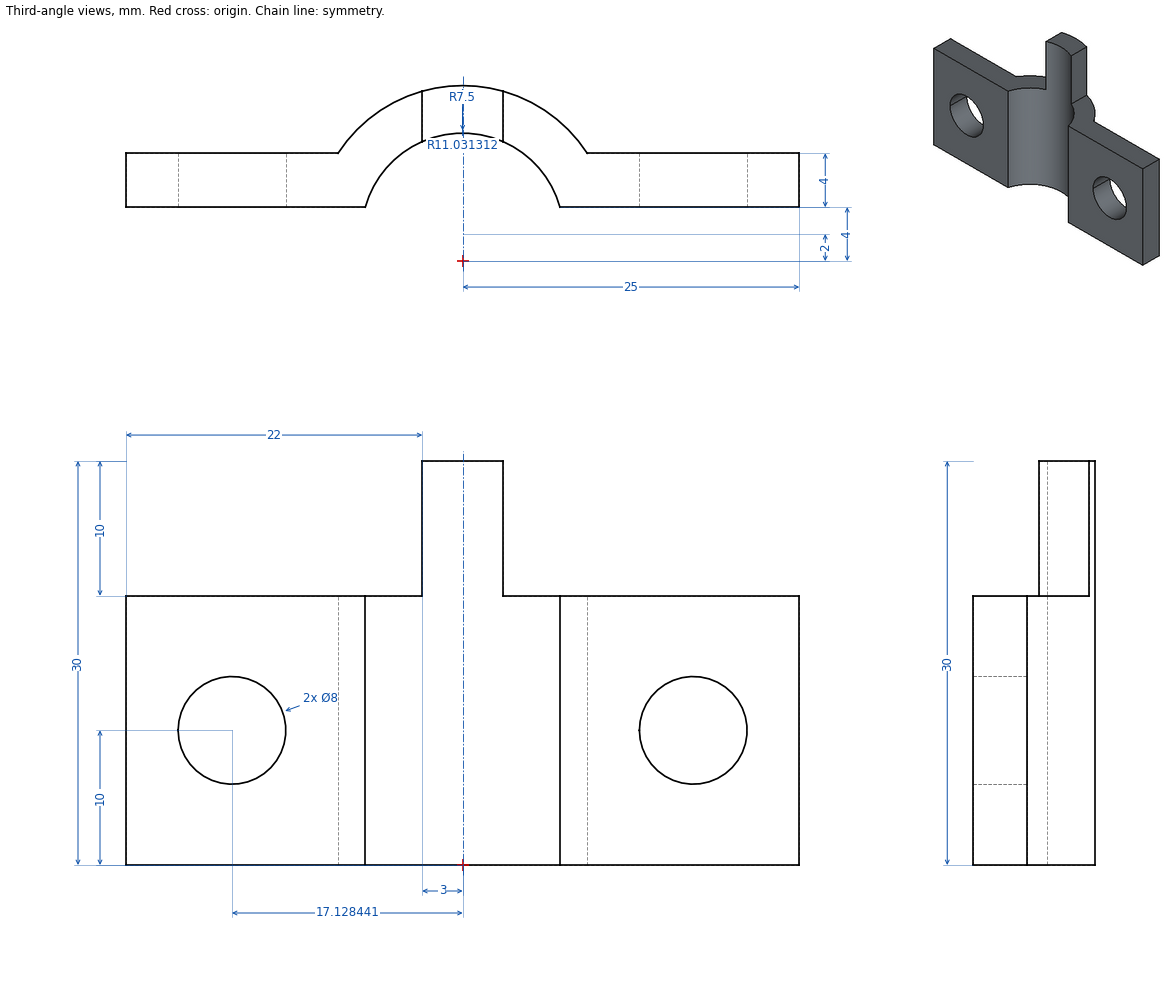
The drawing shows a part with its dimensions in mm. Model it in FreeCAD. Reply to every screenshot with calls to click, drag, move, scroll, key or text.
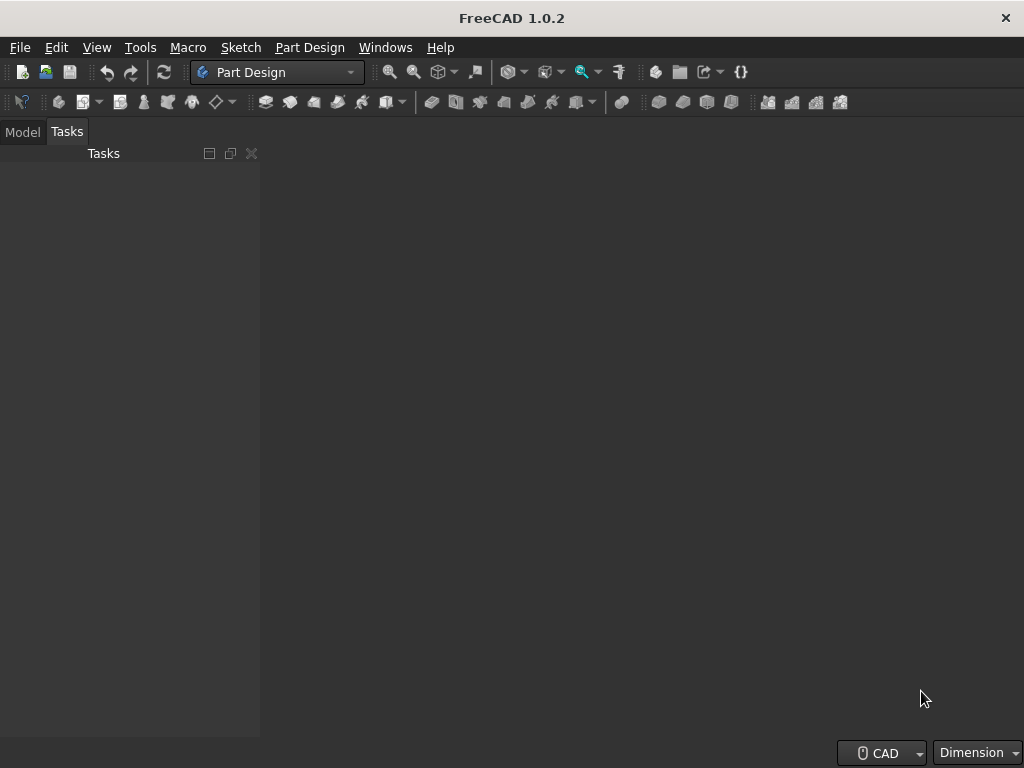
click(574, 102)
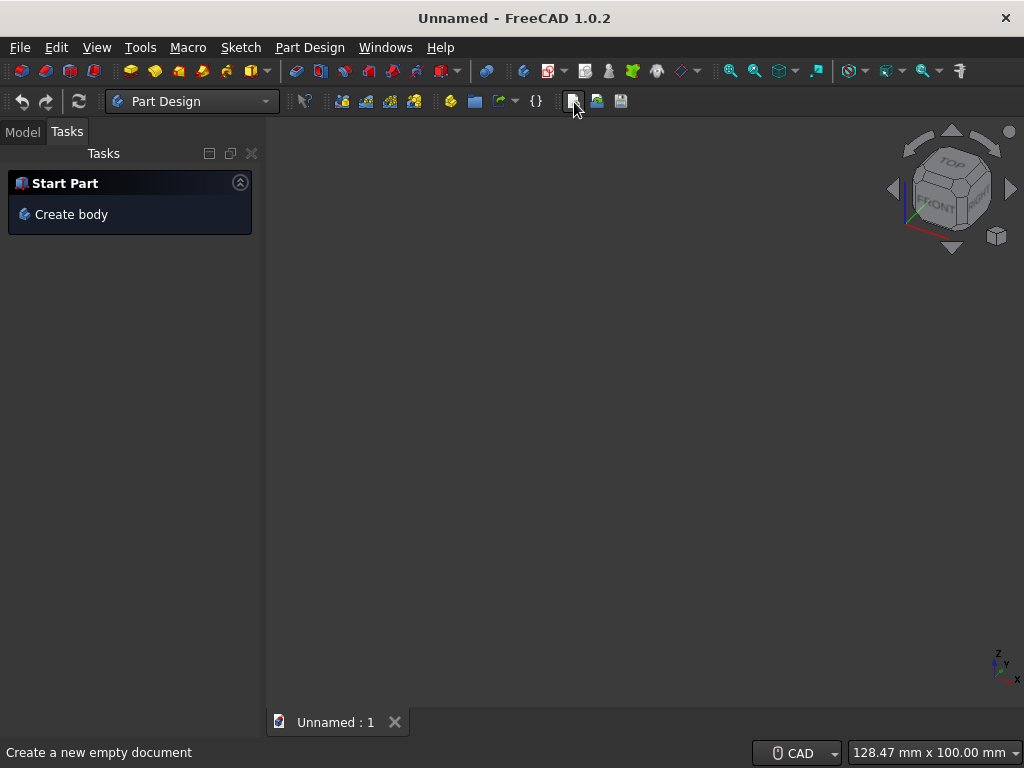
click(548, 72)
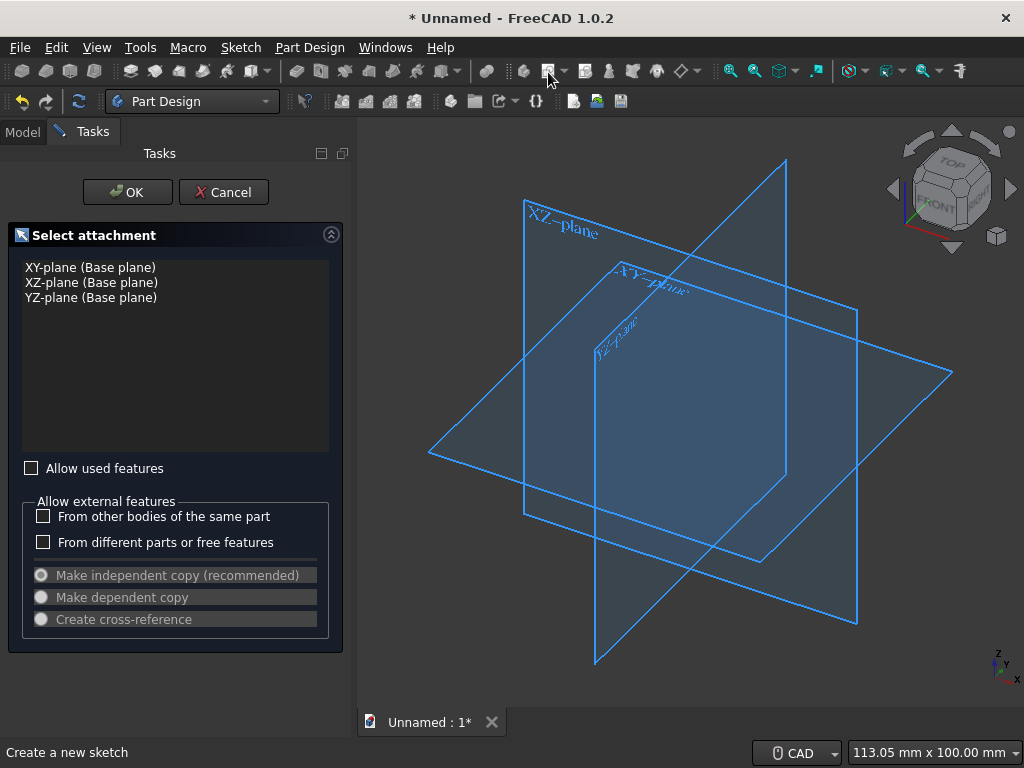
click(82, 268)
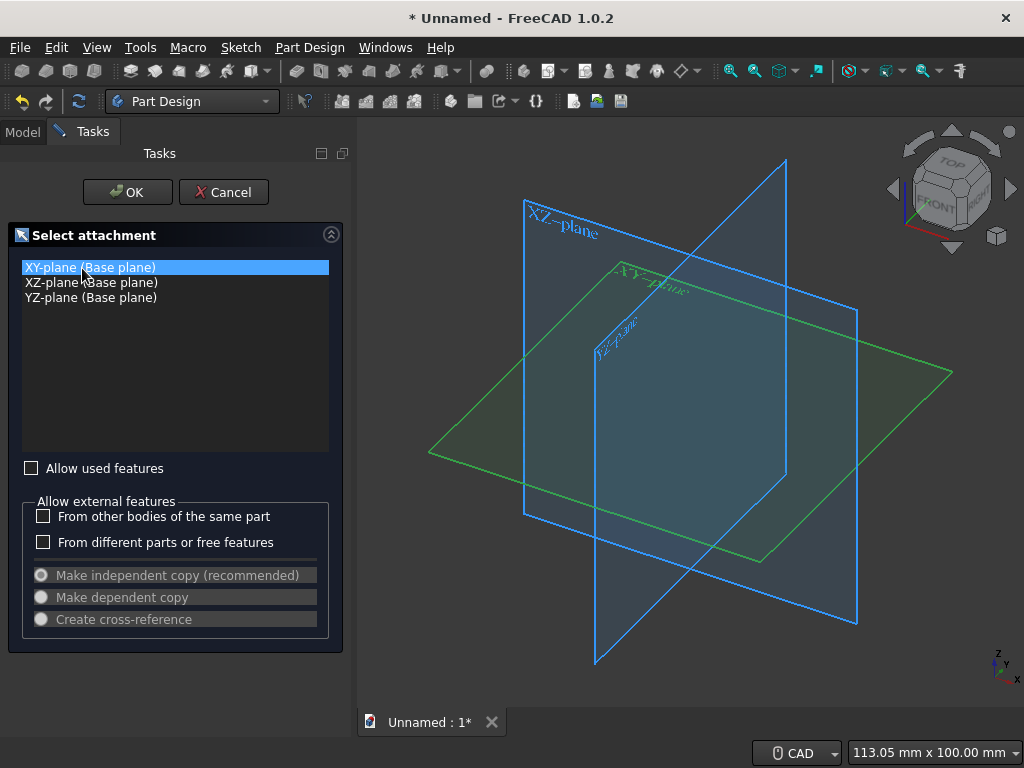
click(128, 192)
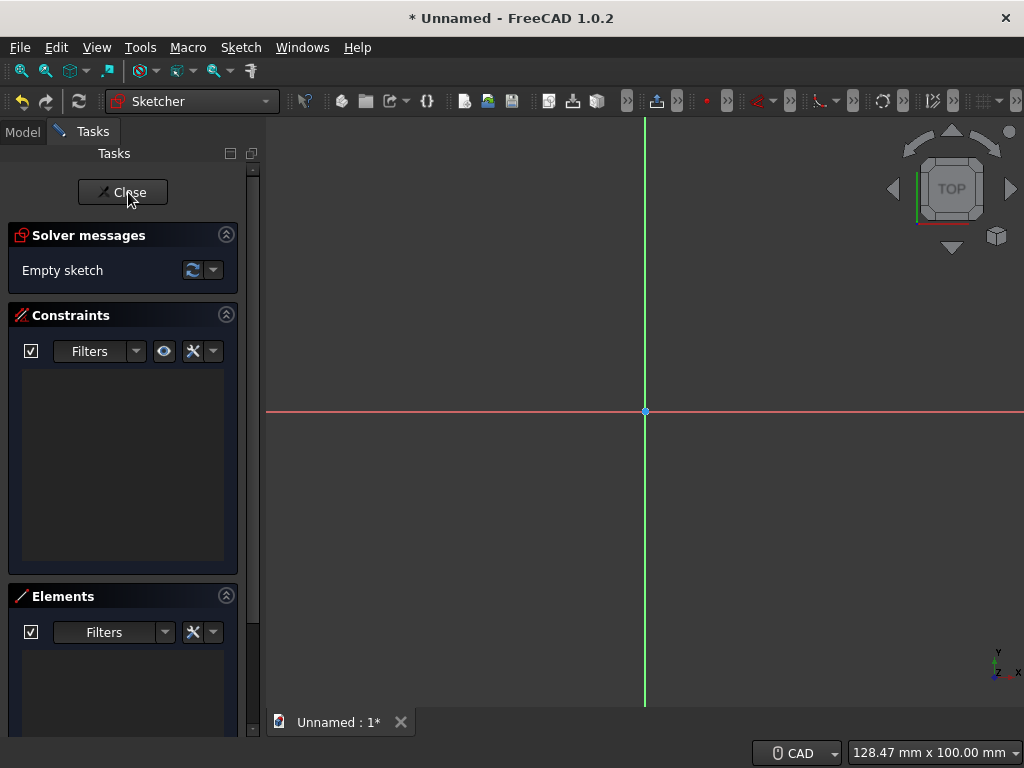
scroll(784, 295, up, 2)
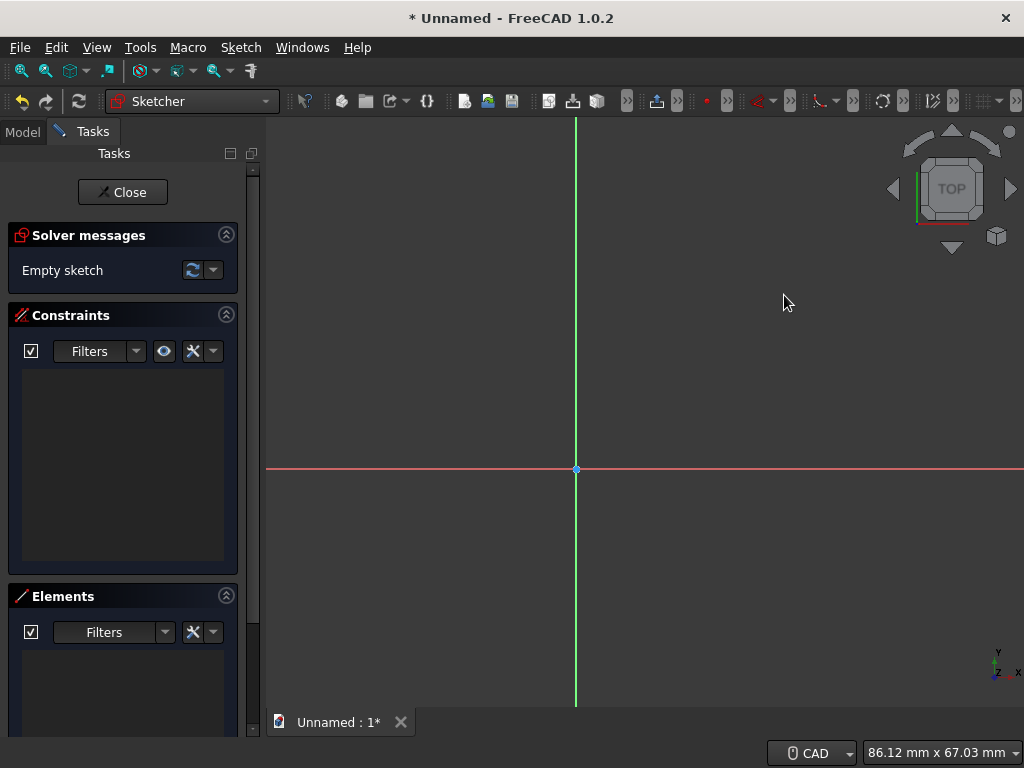
key(g)
key(m)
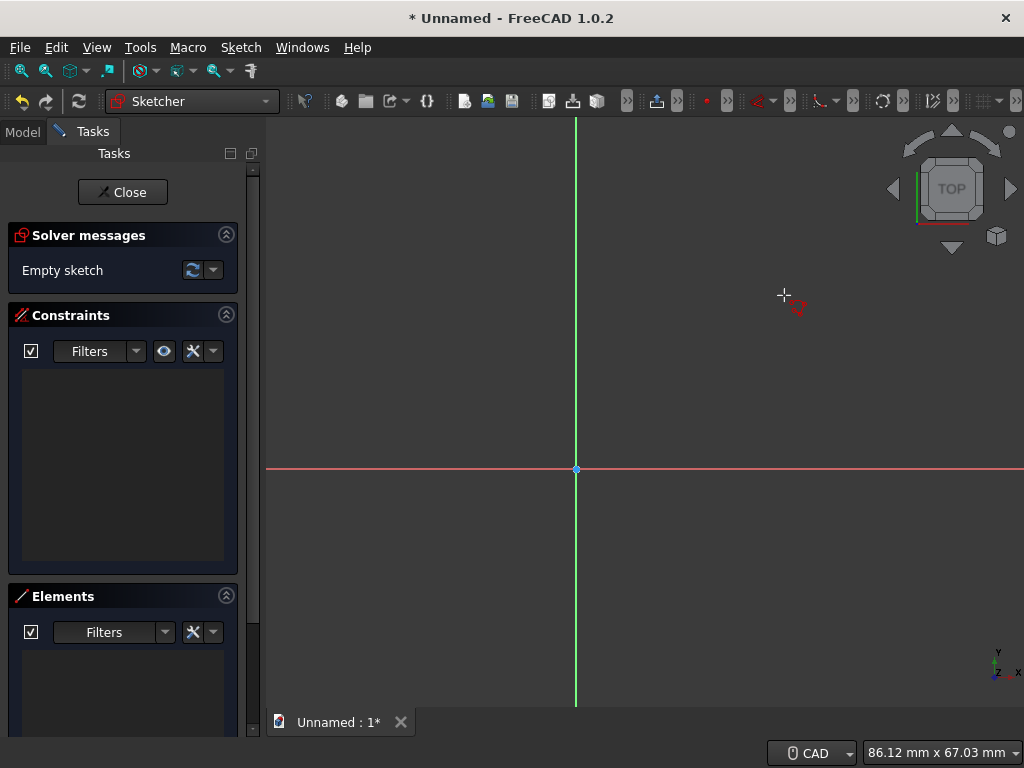
click(640, 434)
click(796, 434)
click(796, 399)
click(658, 399)
right_click(658, 399)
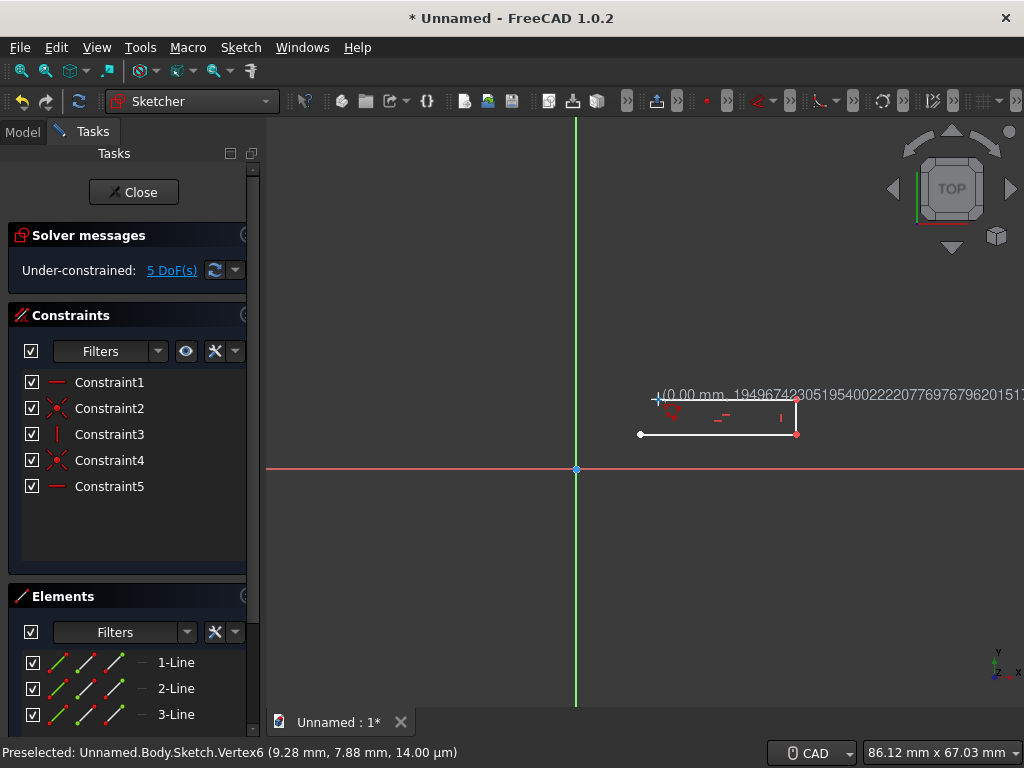
click(495, 399)
click(356, 399)
click(356, 434)
click(513, 434)
right_click(513, 434)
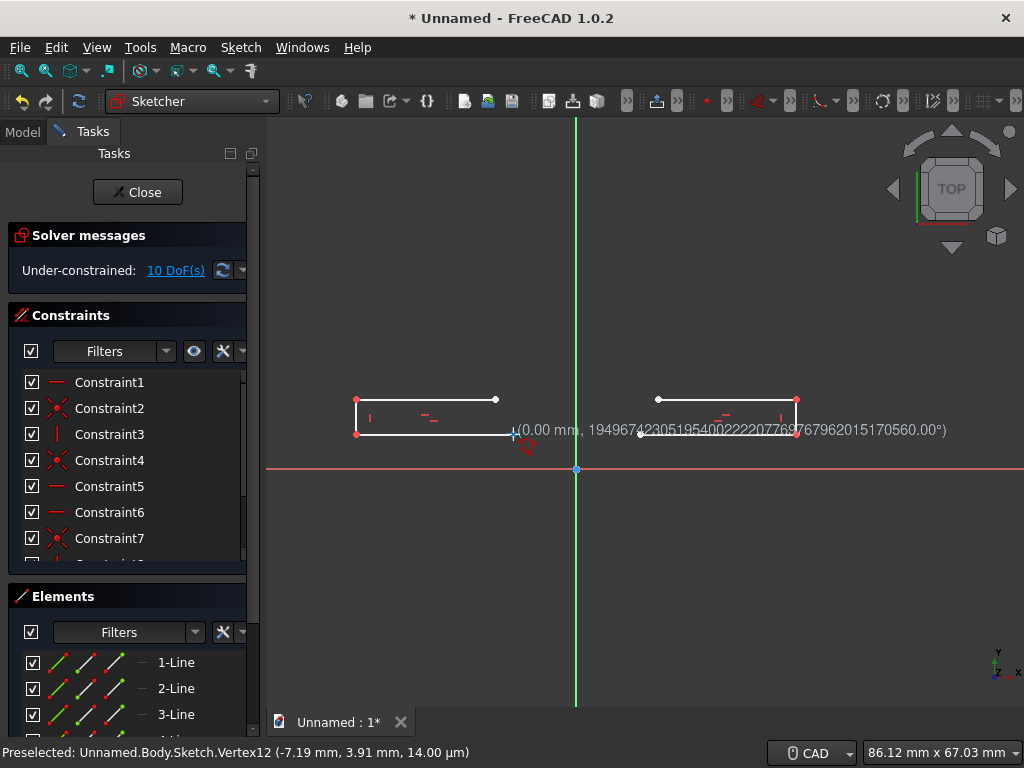
key(g)
key(3)
key(a)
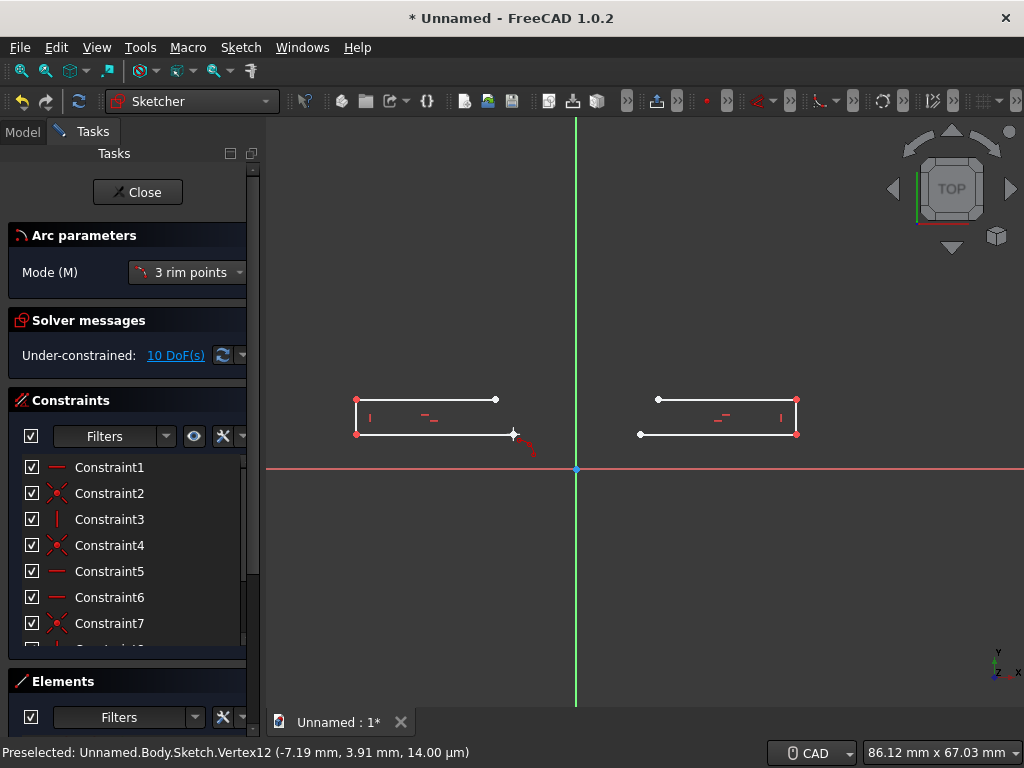
click(658, 400)
click(495, 400)
click(596, 357)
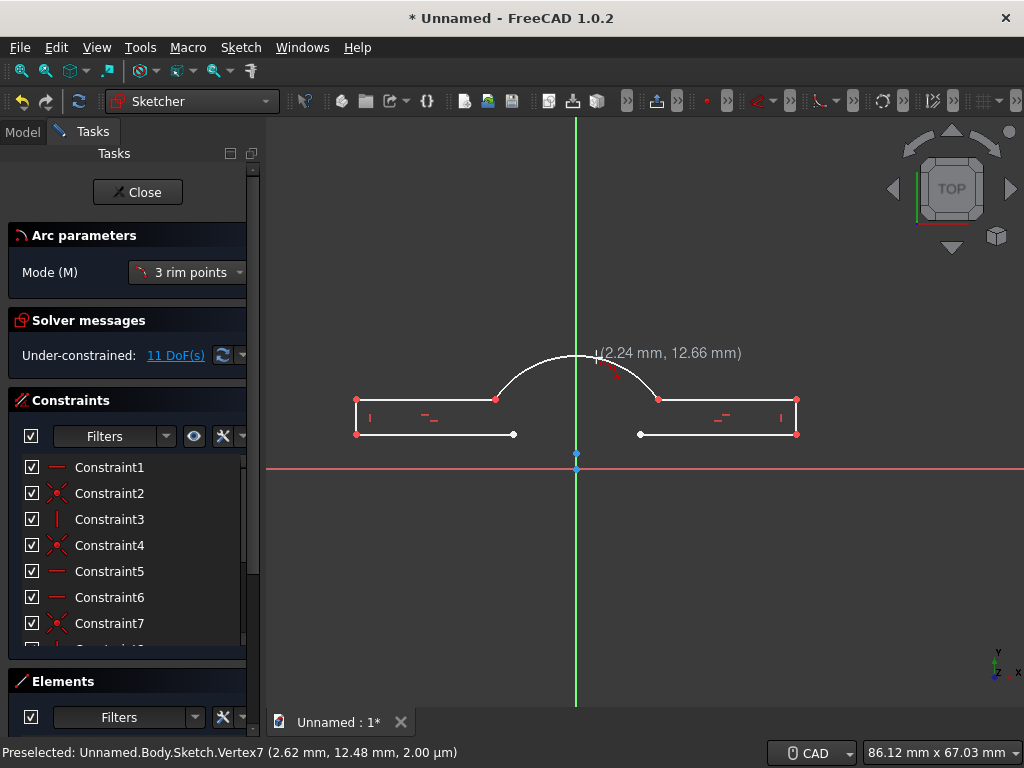
click(513, 435)
click(640, 435)
click(593, 388)
key(Escape)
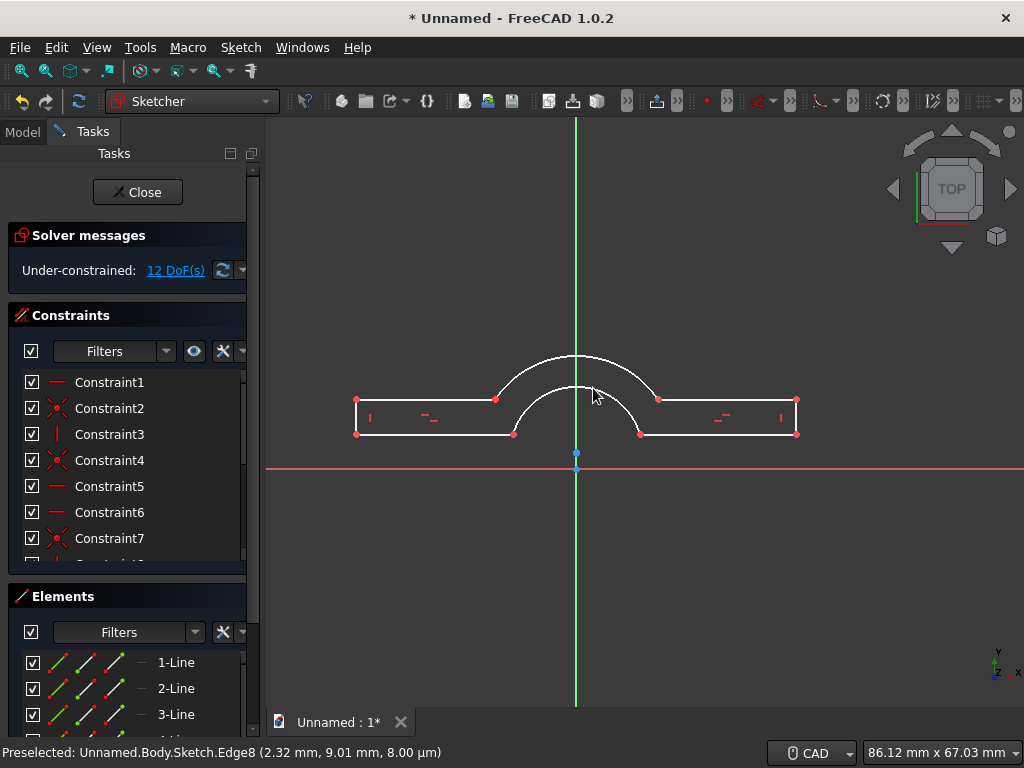
click(614, 364)